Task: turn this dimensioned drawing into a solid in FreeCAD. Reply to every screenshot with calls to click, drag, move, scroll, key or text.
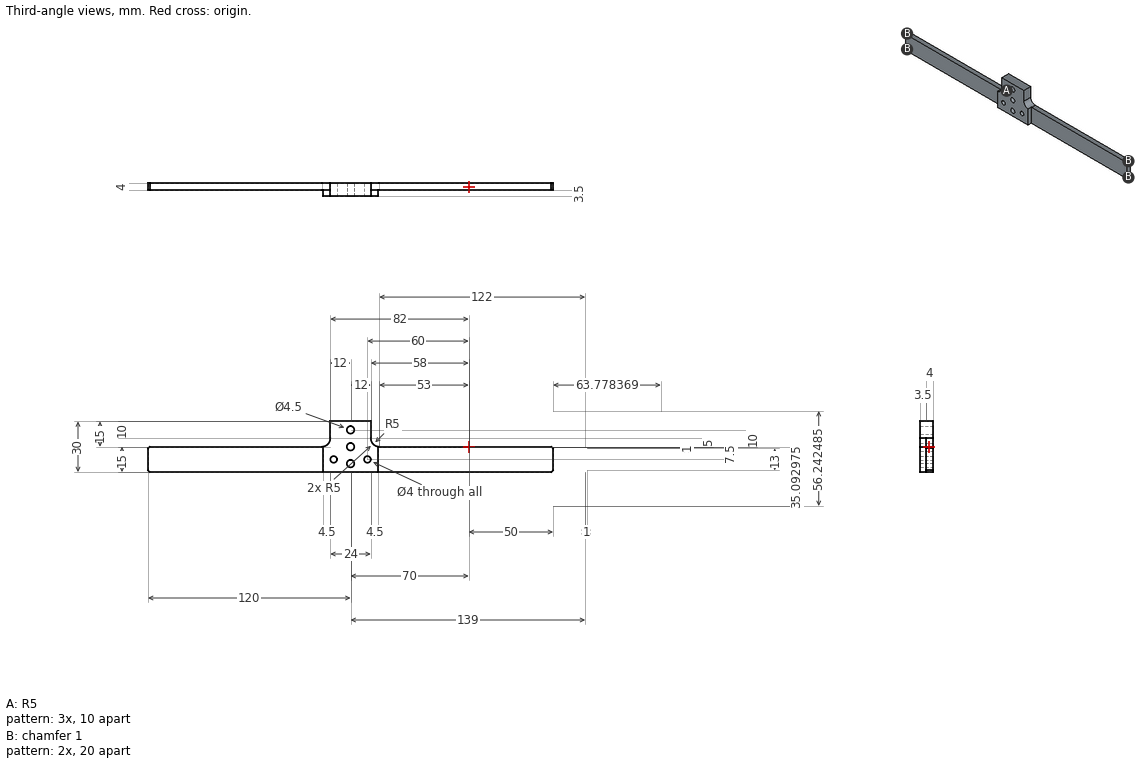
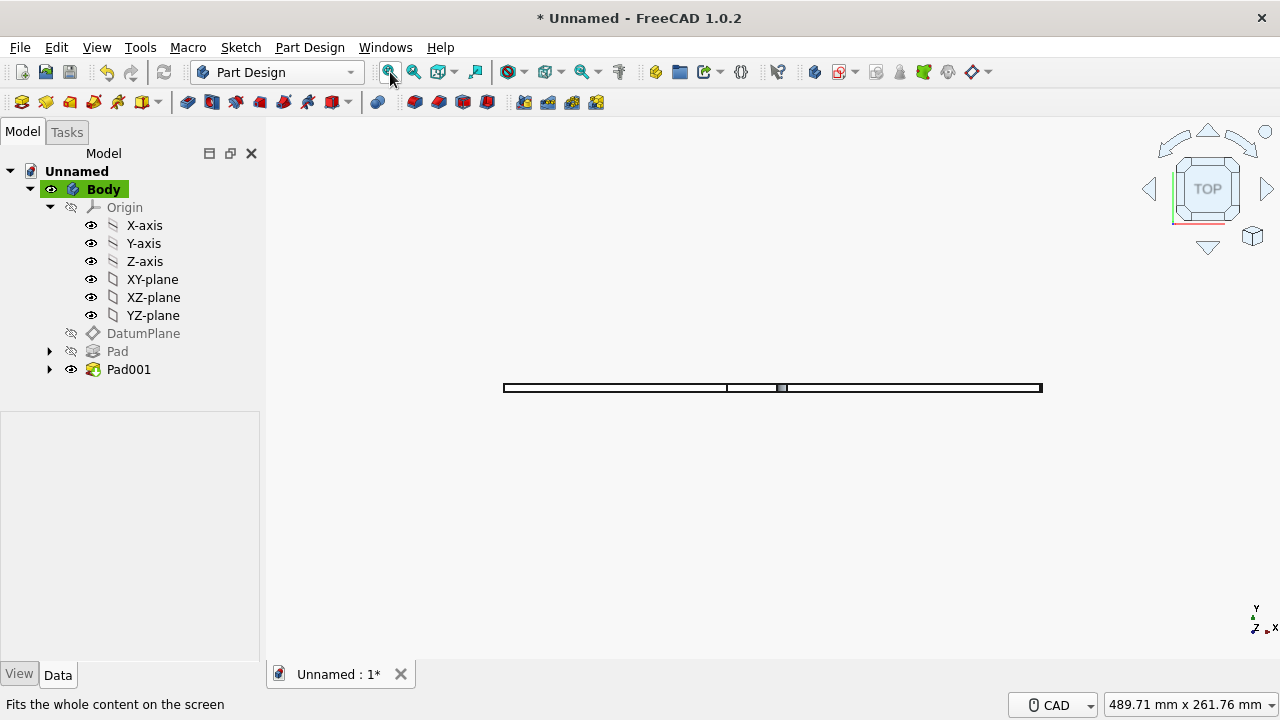
key(1)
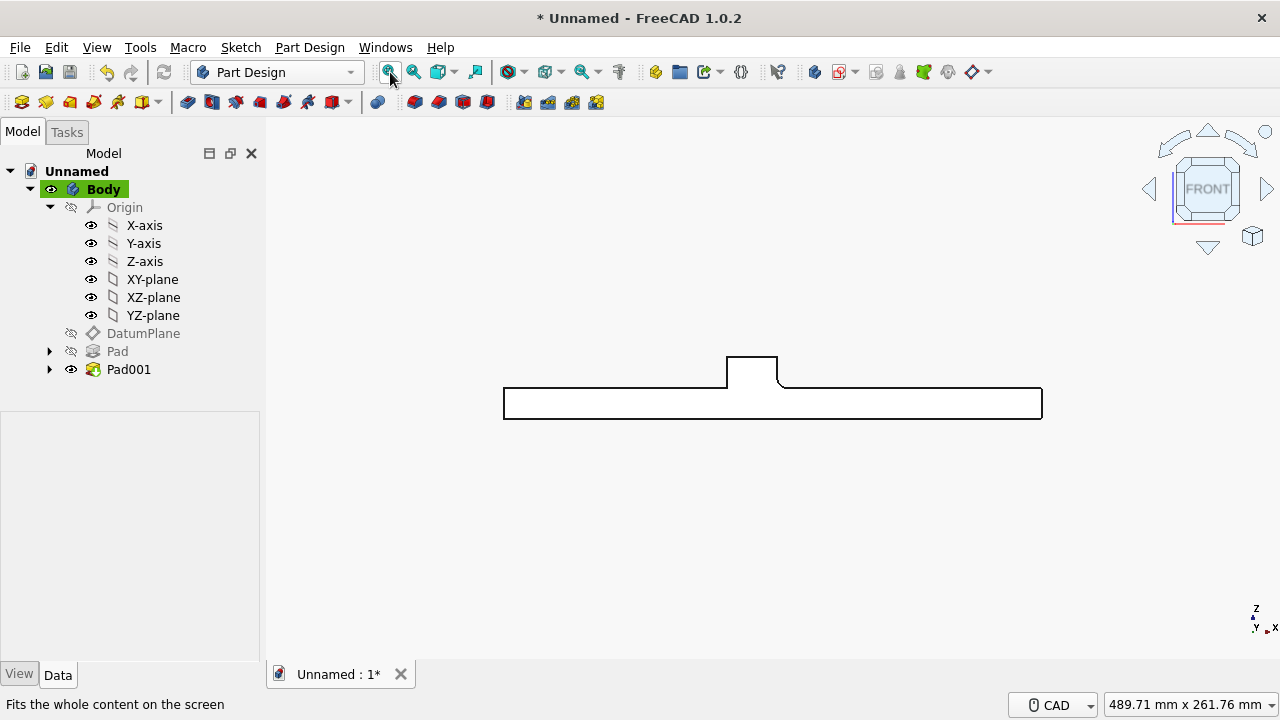
scroll(727, 387, up, 8)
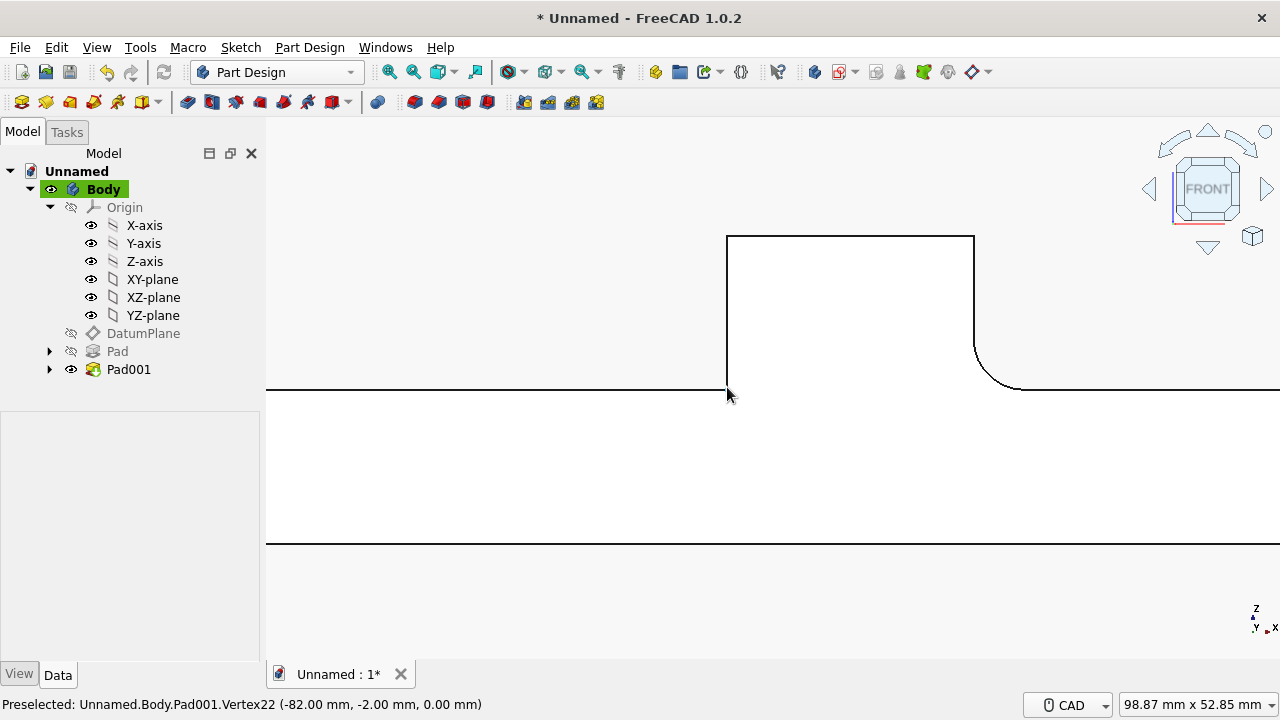
click(390, 72)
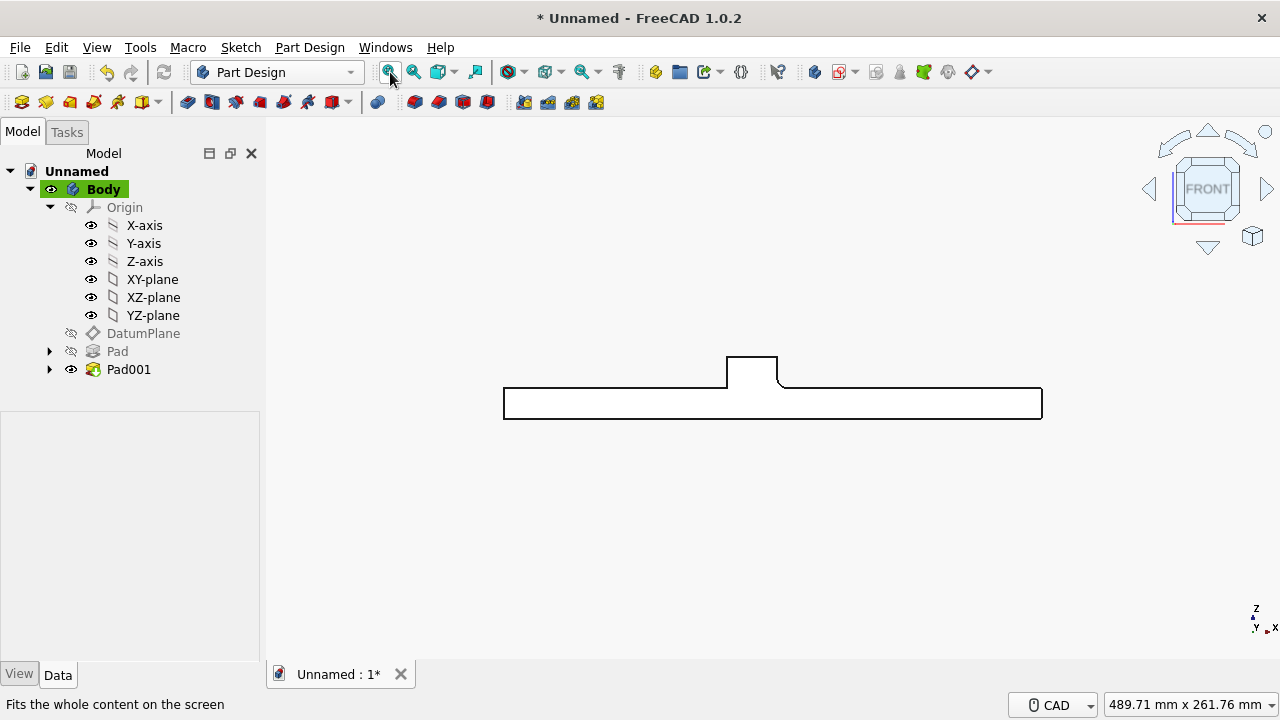
key(3)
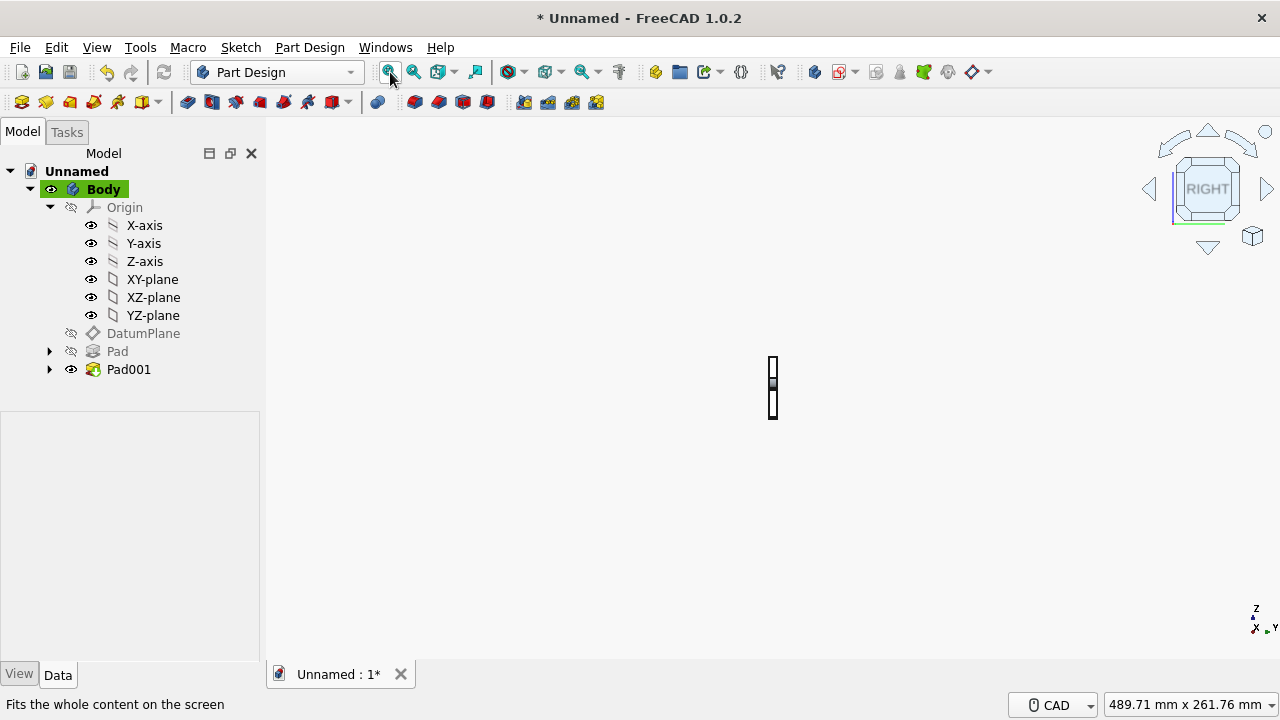
click(390, 72)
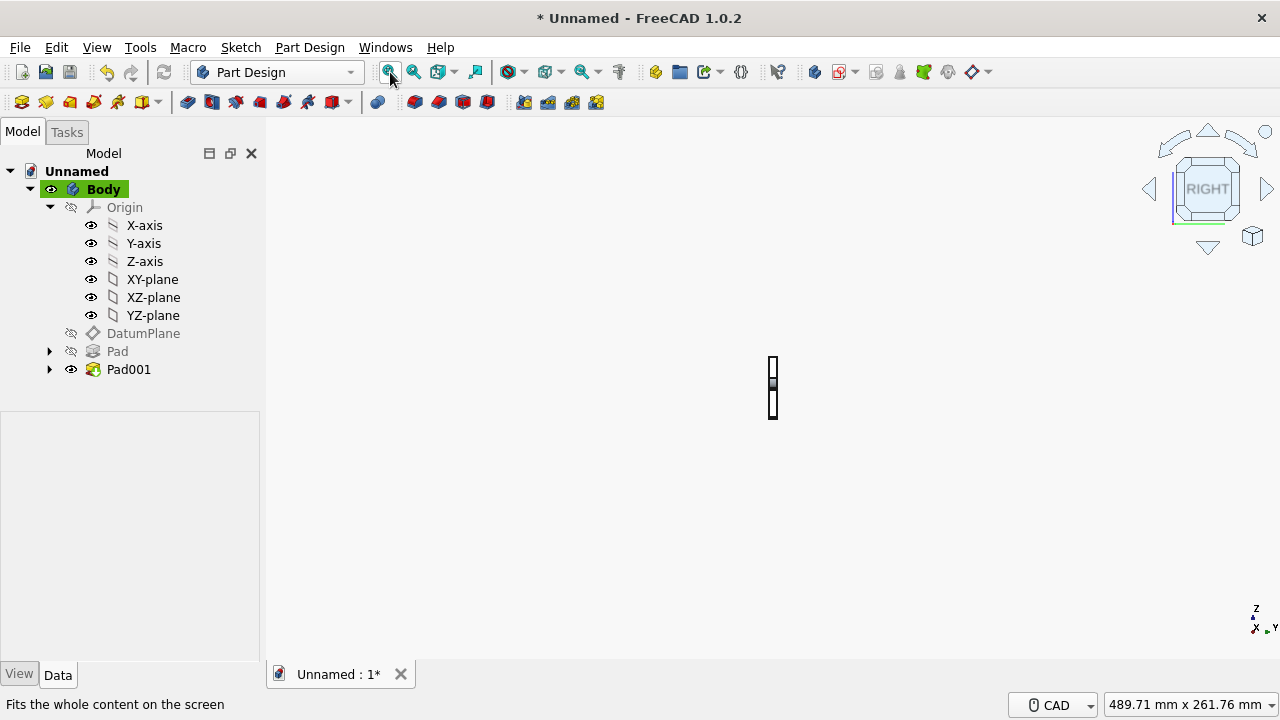
scroll(773, 387, up, 8)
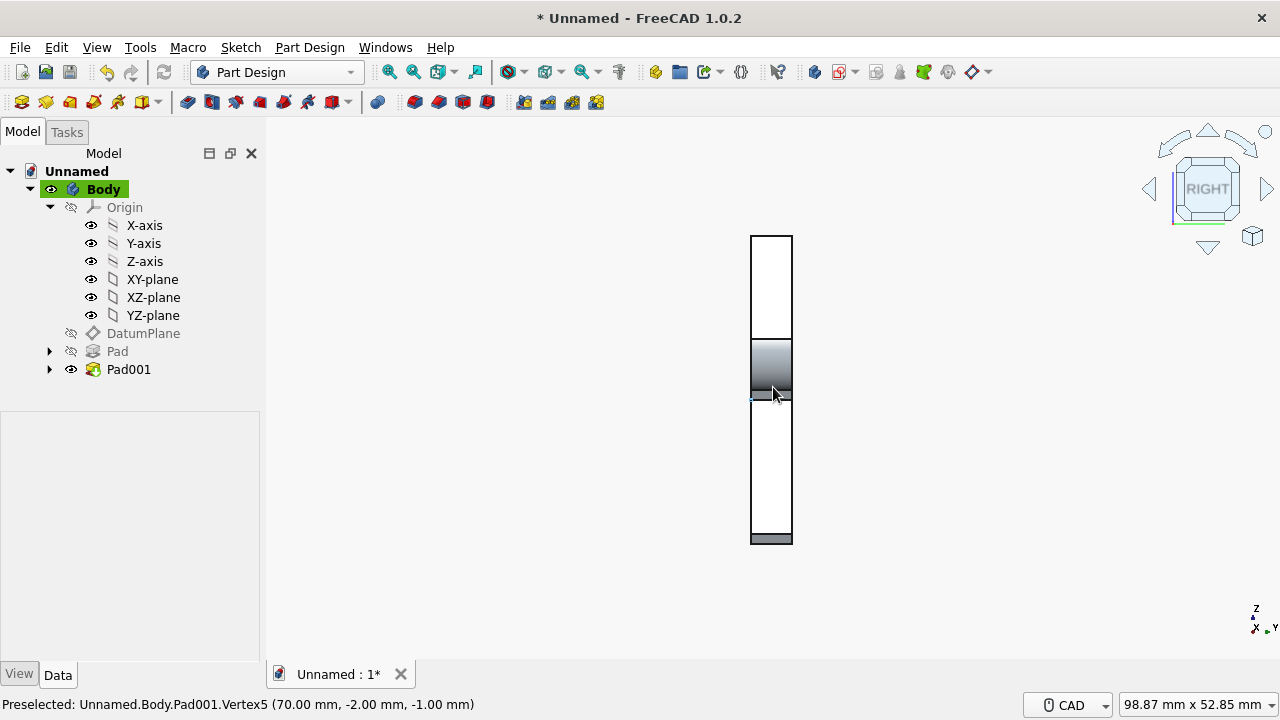
click(390, 72)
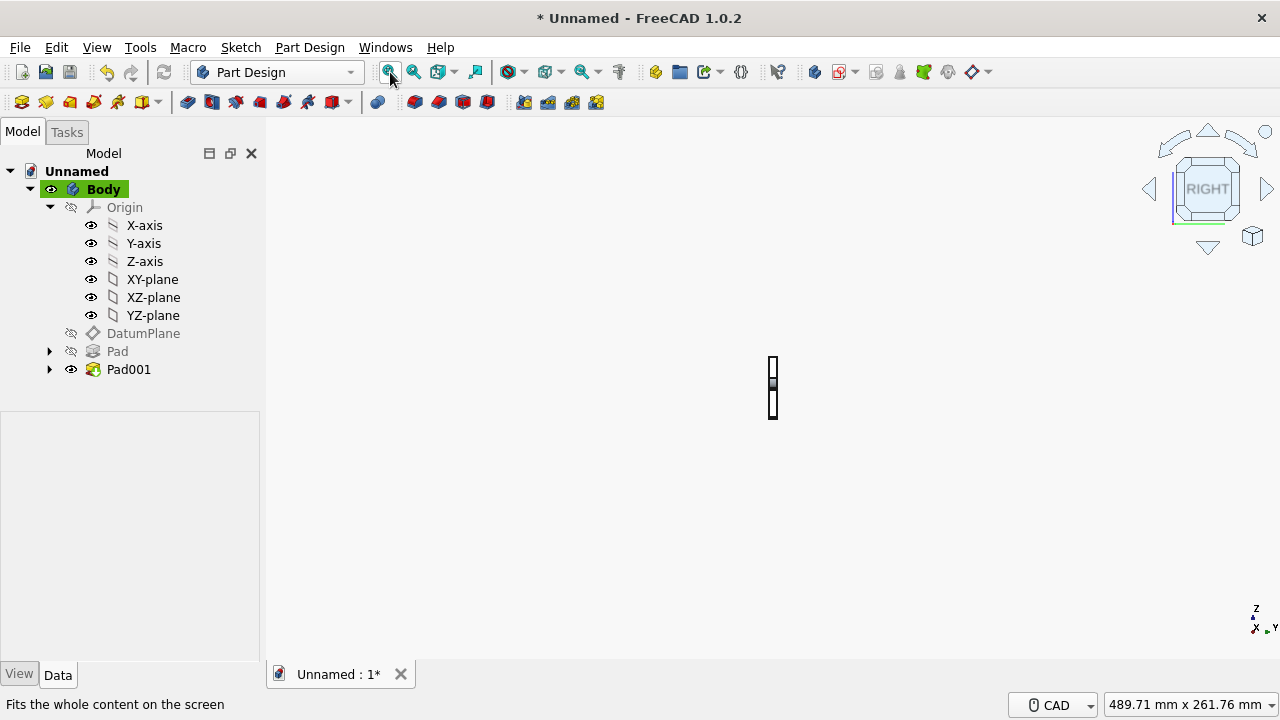
key(5)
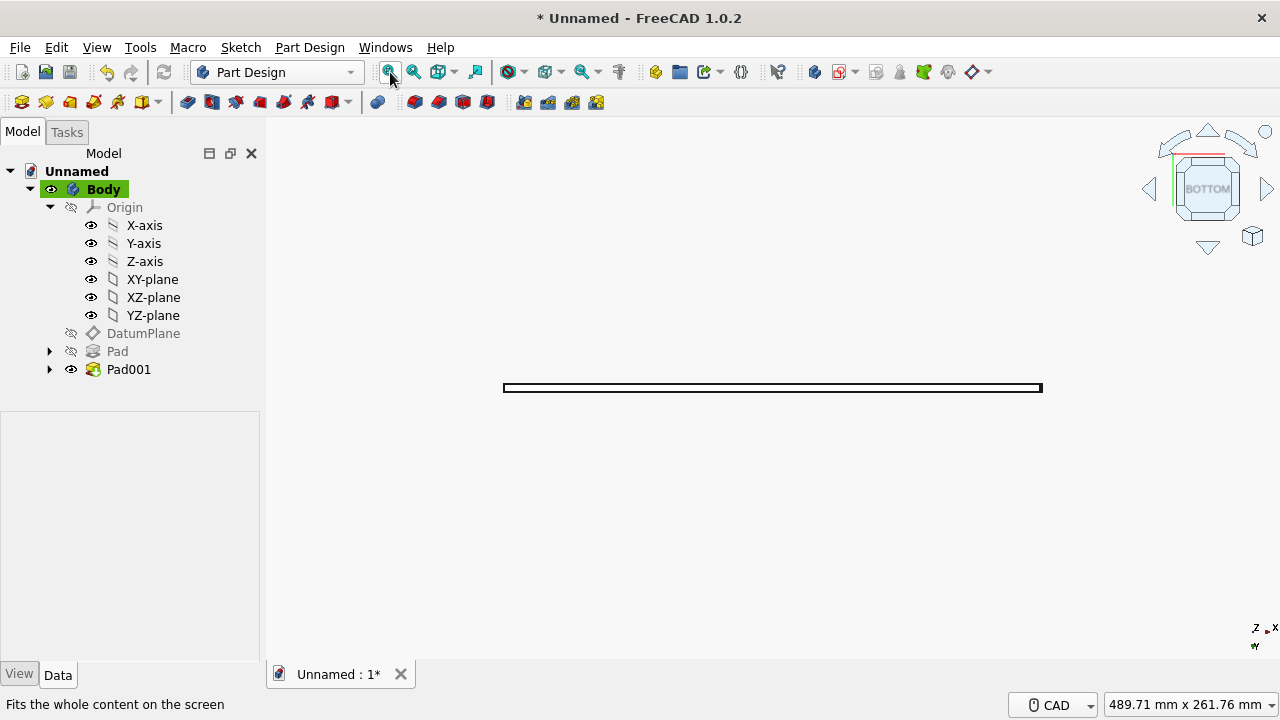
scroll(727, 387, up, 8)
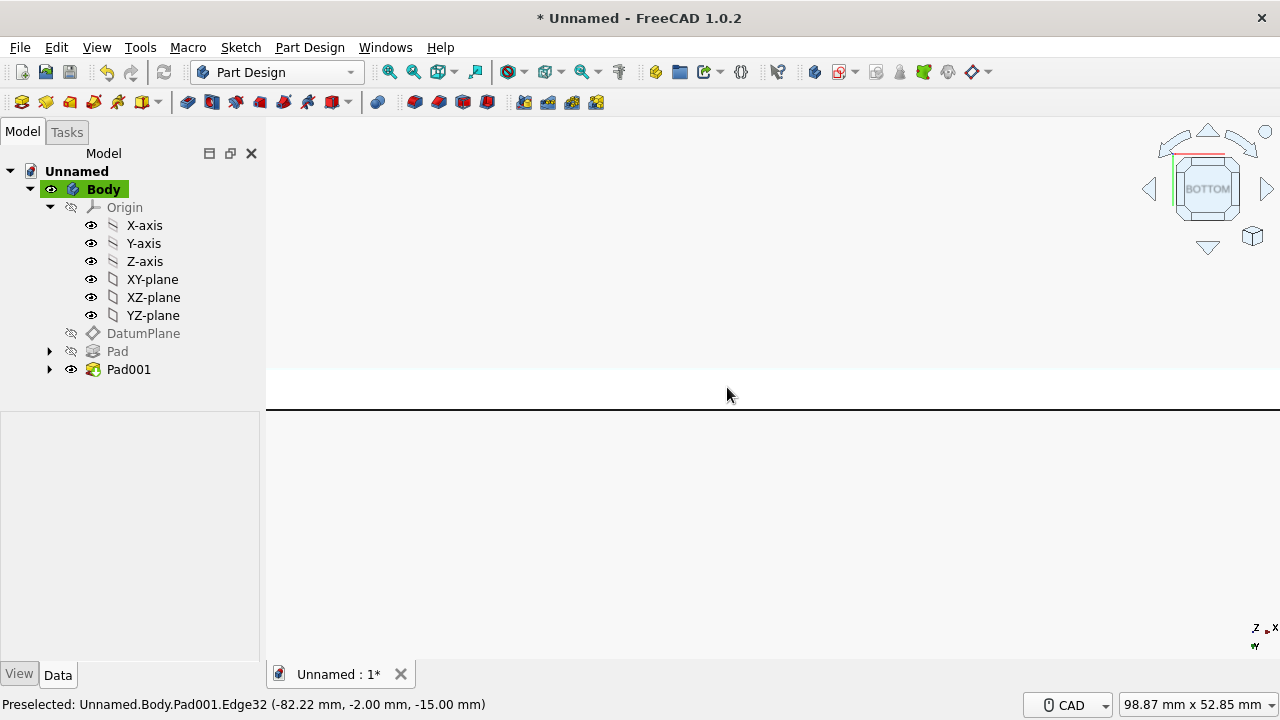
click(390, 72)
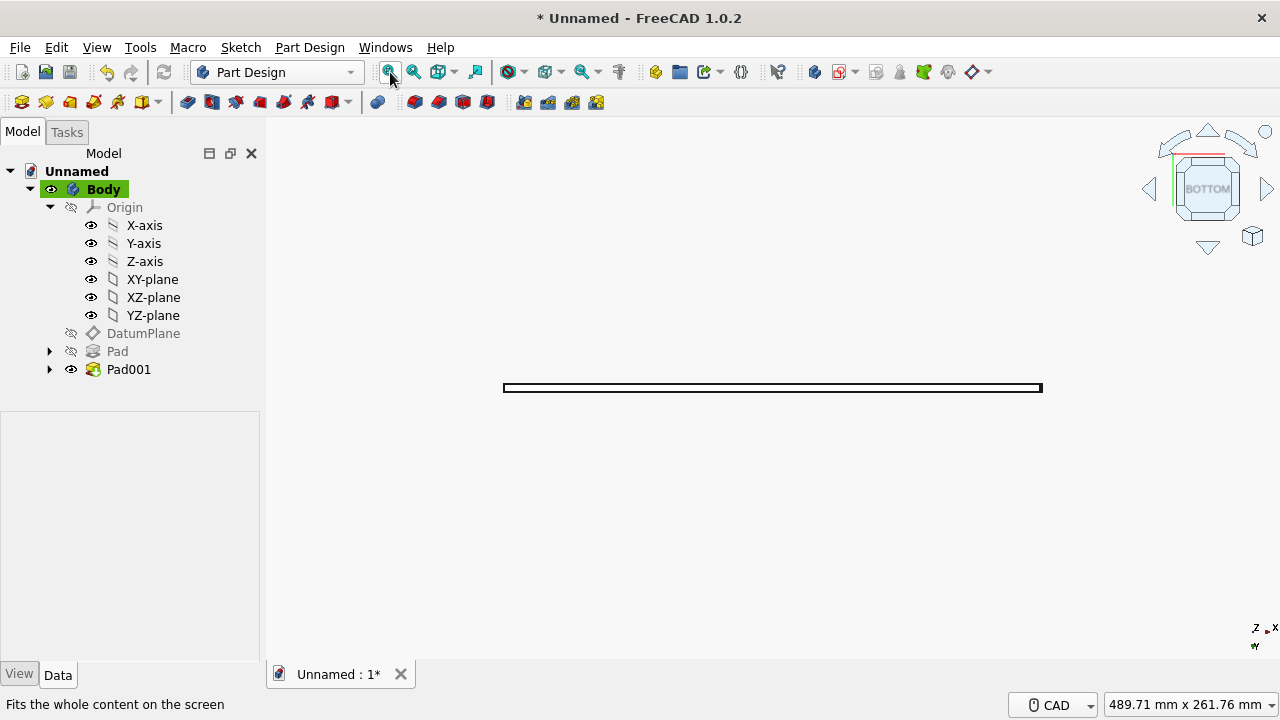
key(4)